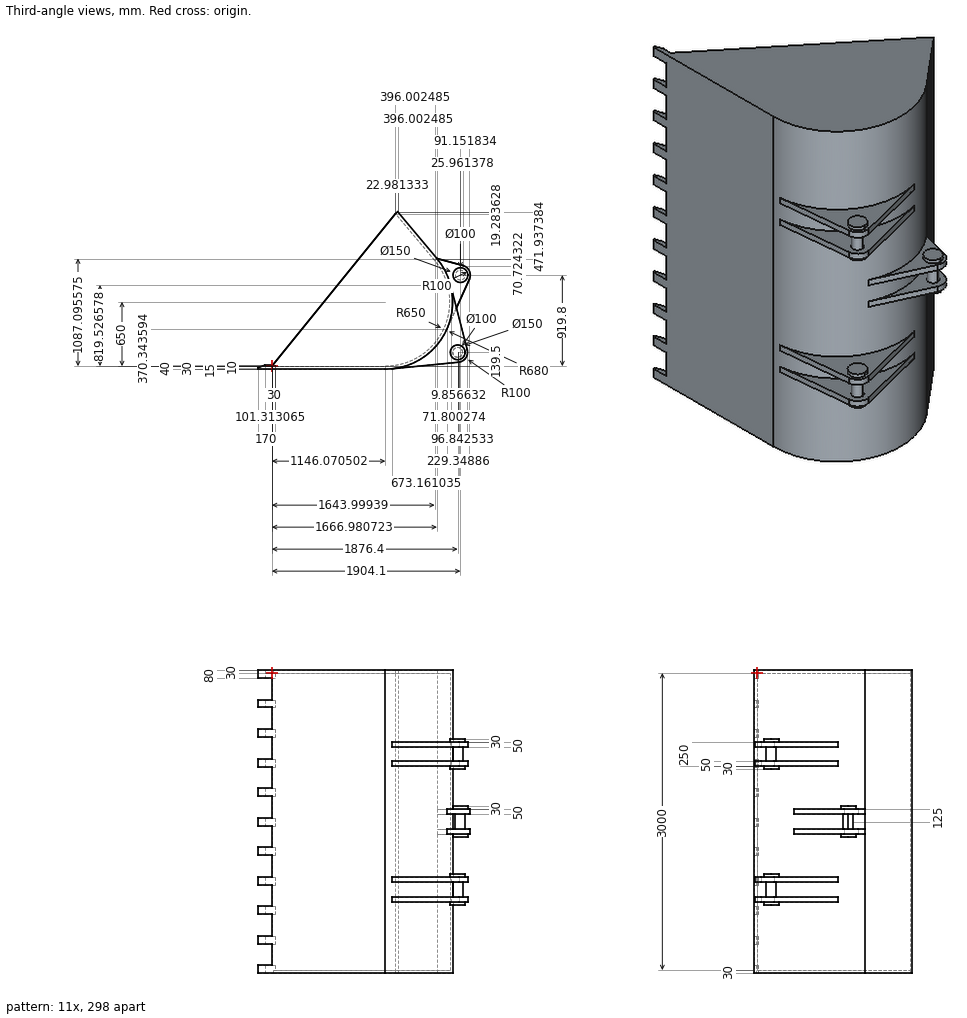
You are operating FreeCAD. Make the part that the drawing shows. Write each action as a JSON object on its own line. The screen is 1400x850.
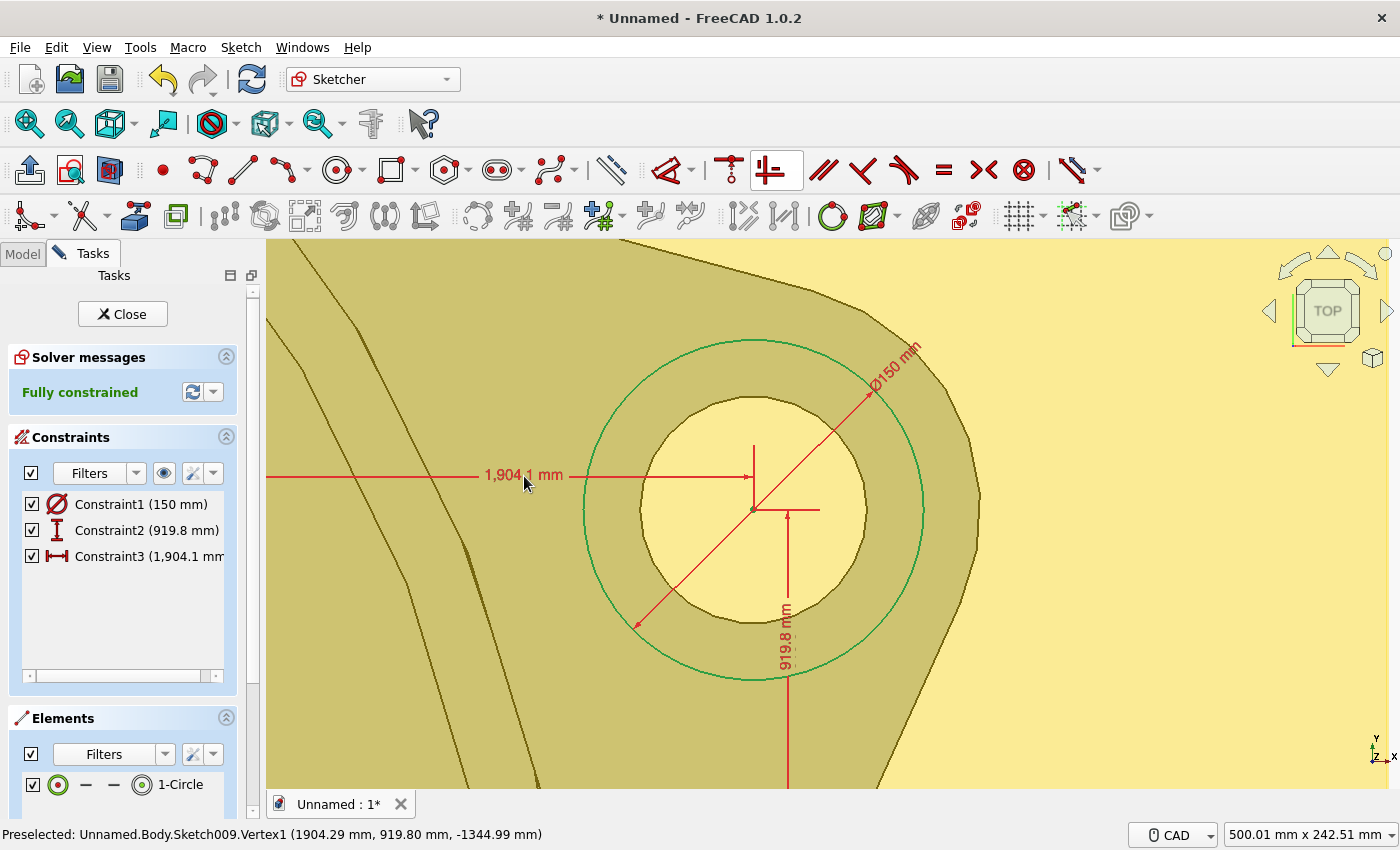
{"action": "left_click", "coordinate": [123, 314]}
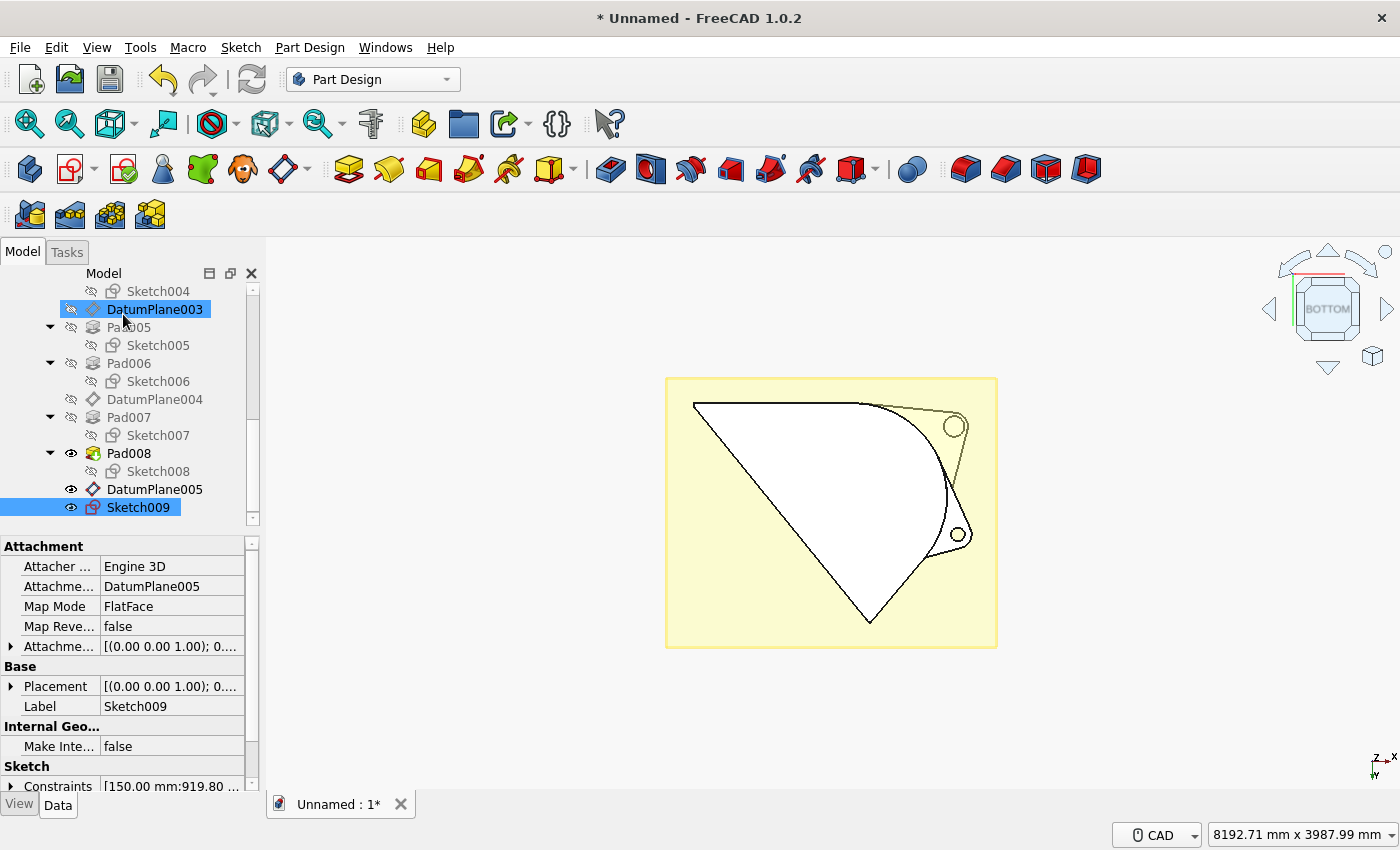
{"action": "left_click", "coordinate": [350, 170]}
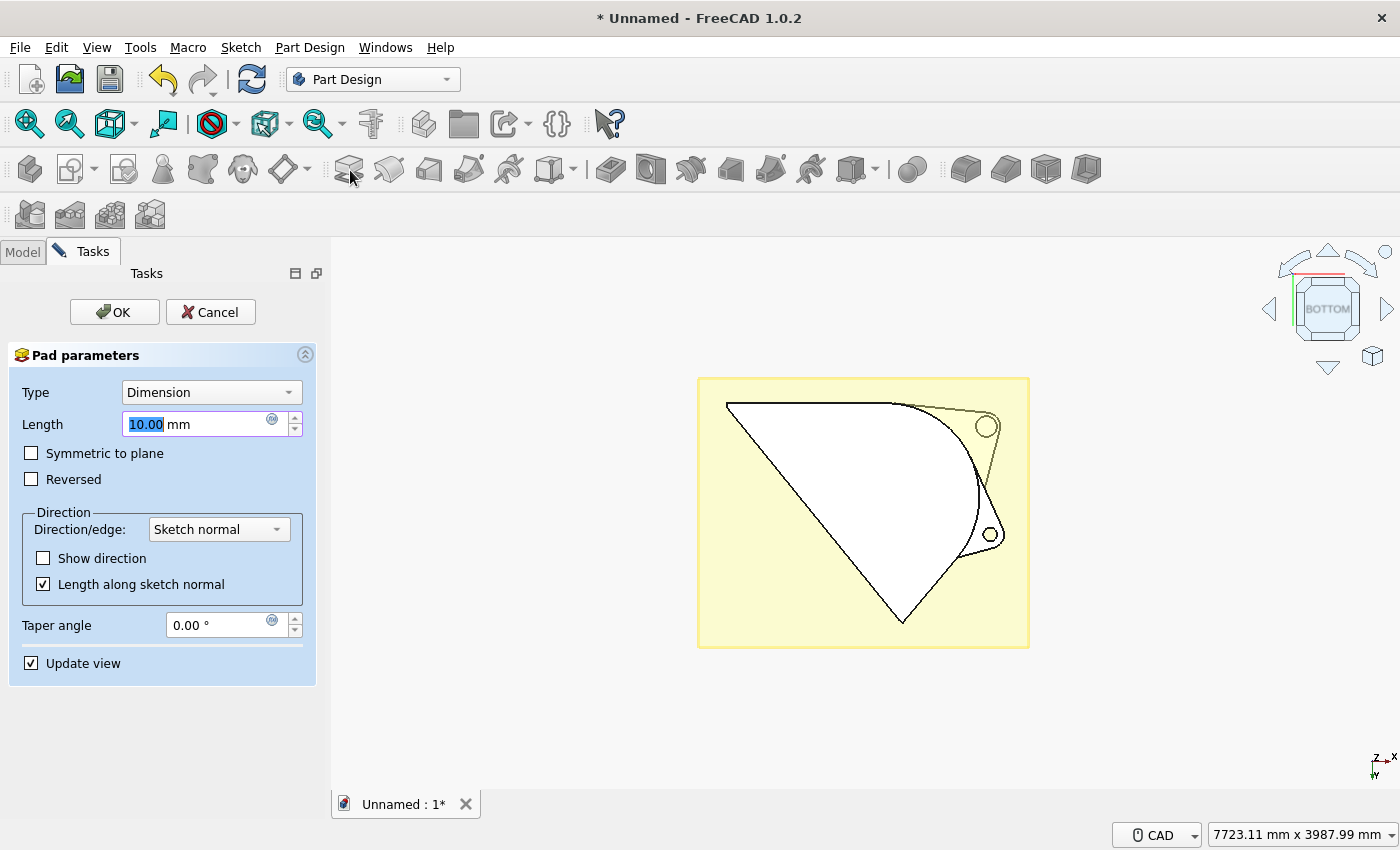
{"action": "type", "text": "30"}
{"action": "key", "text": "Tab"}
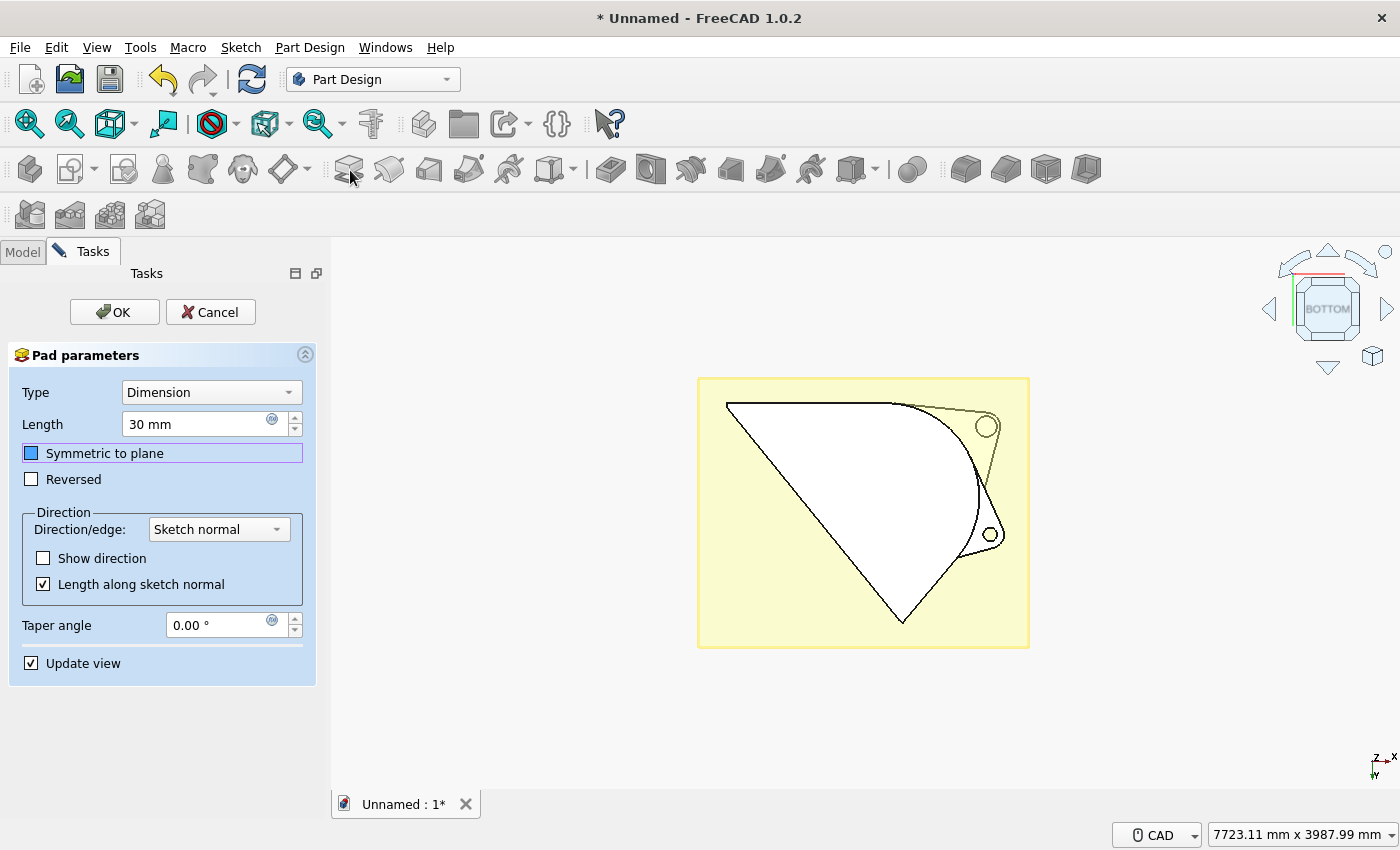
{"action": "left_click", "coordinate": [30, 479]}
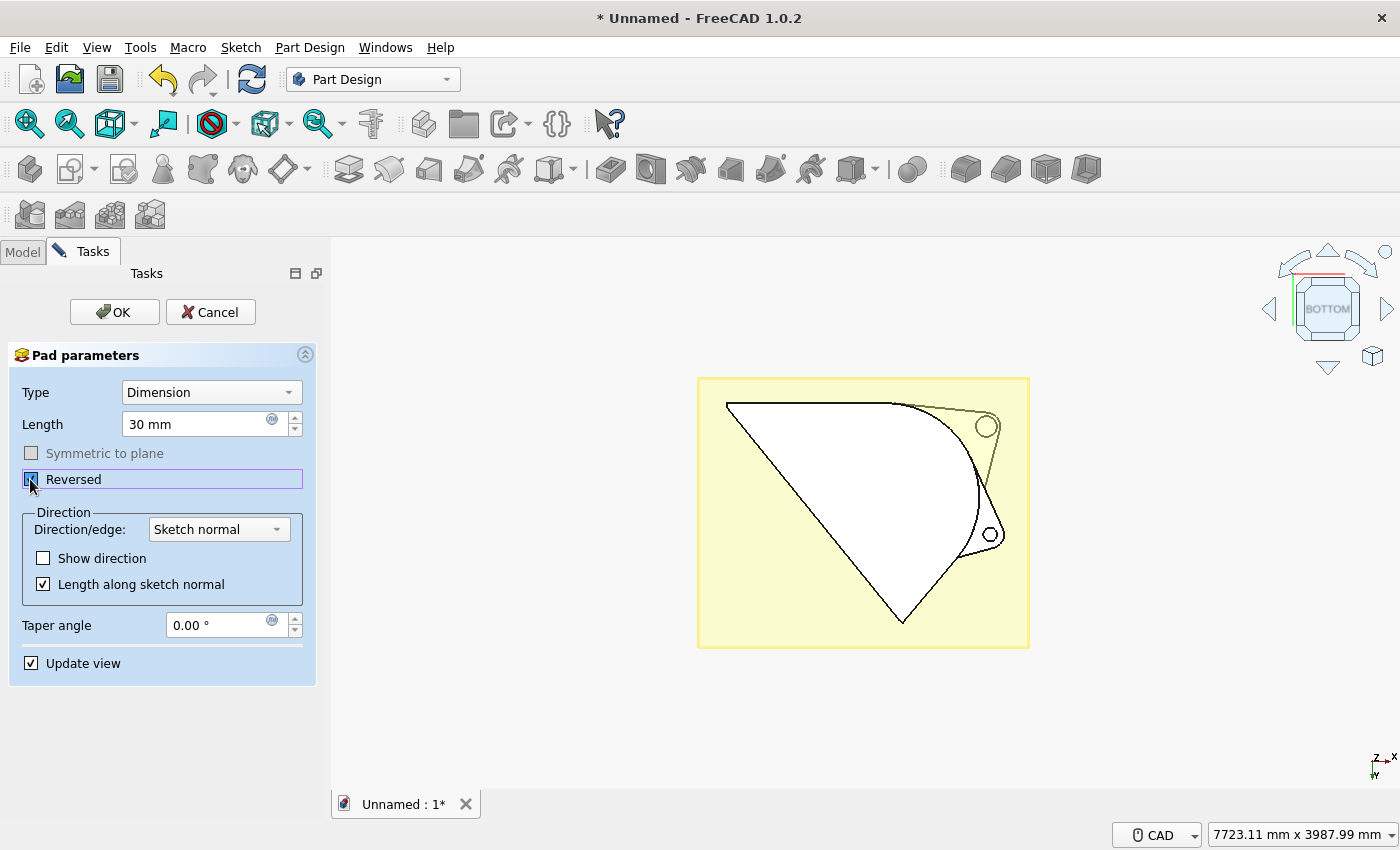
{"action": "left_click", "coordinate": [115, 312]}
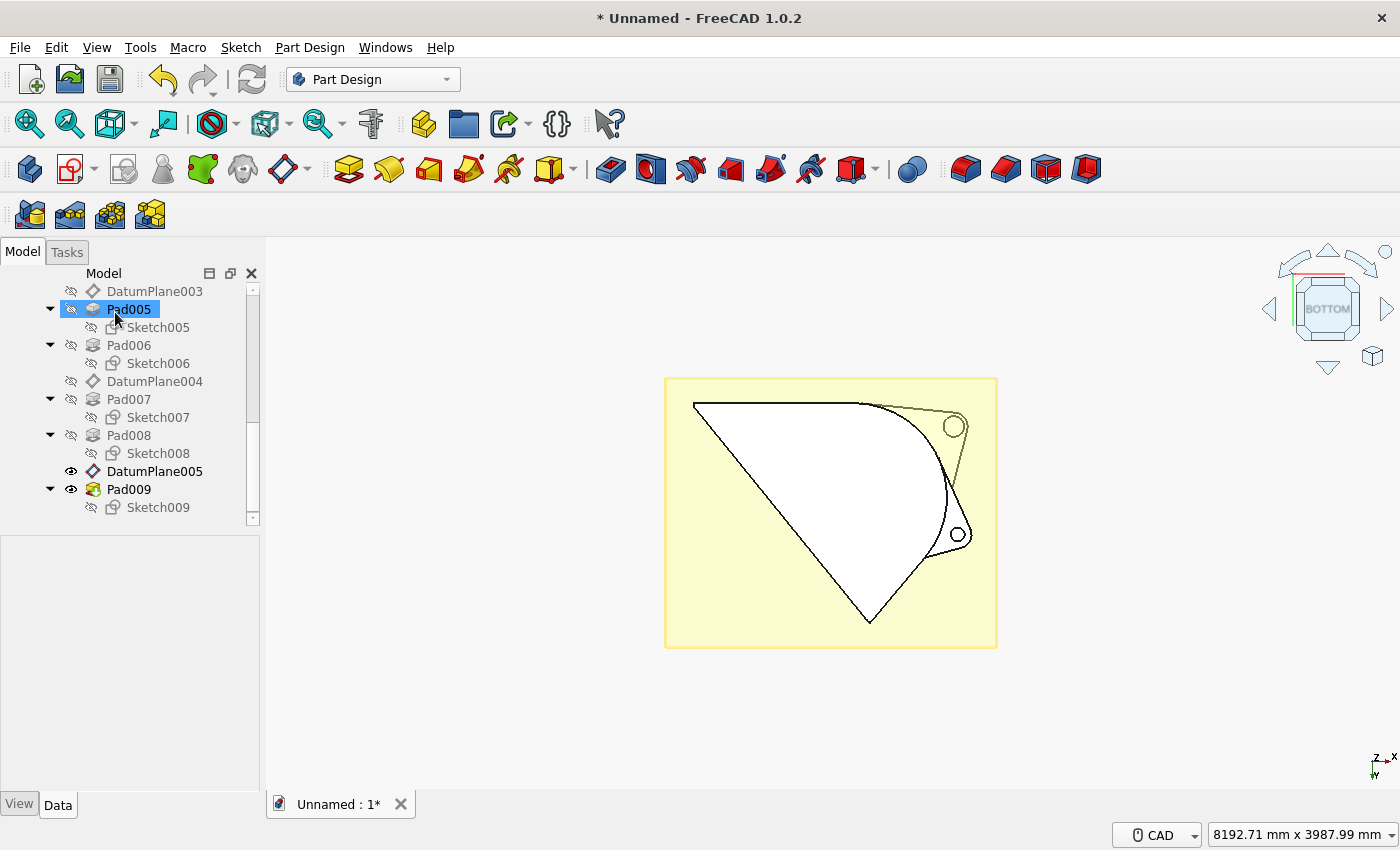
{"action": "left_click", "coordinate": [116, 471]}
{"action": "key", "text": "space"}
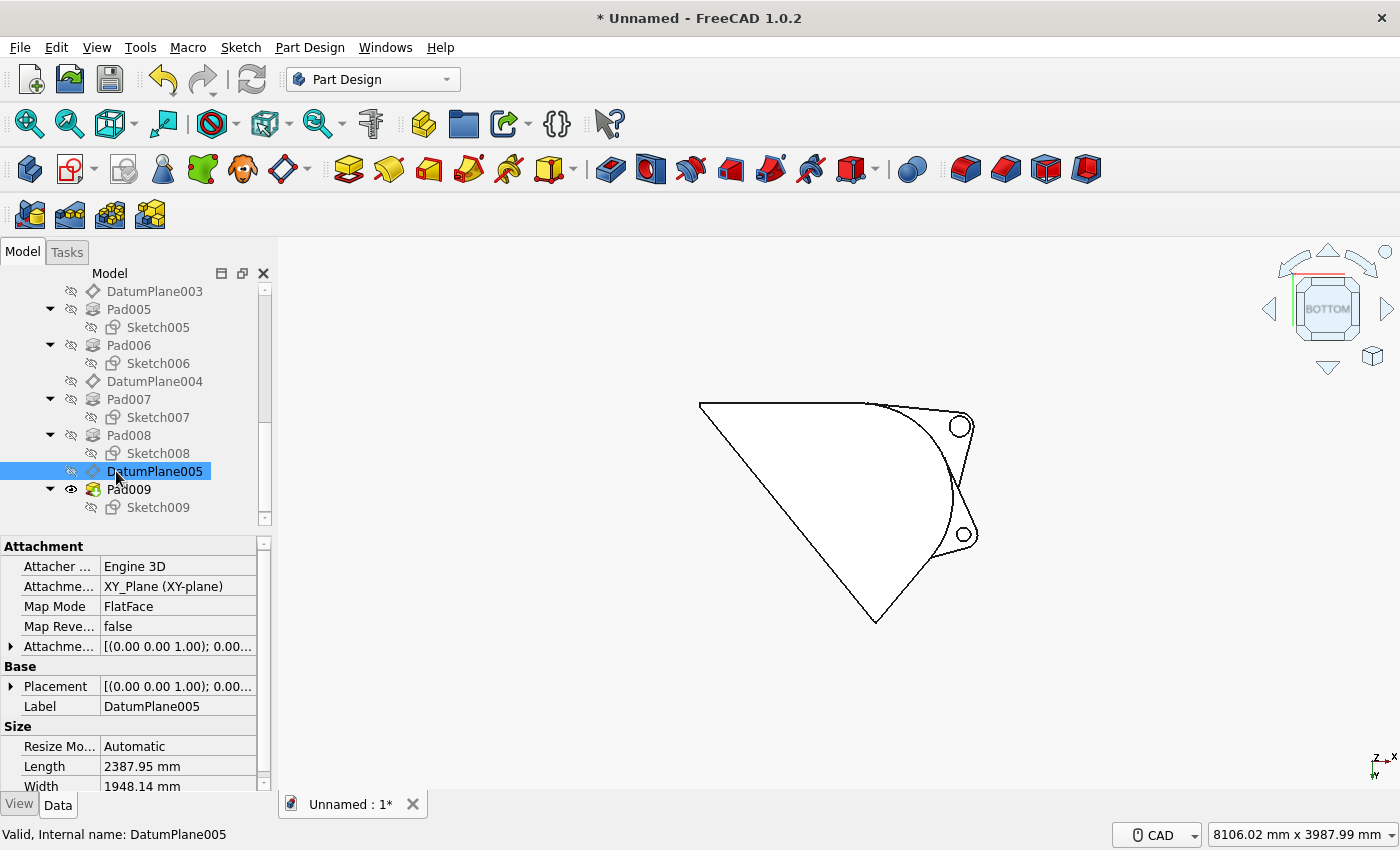
{"action": "left_click", "coordinate": [30, 124]}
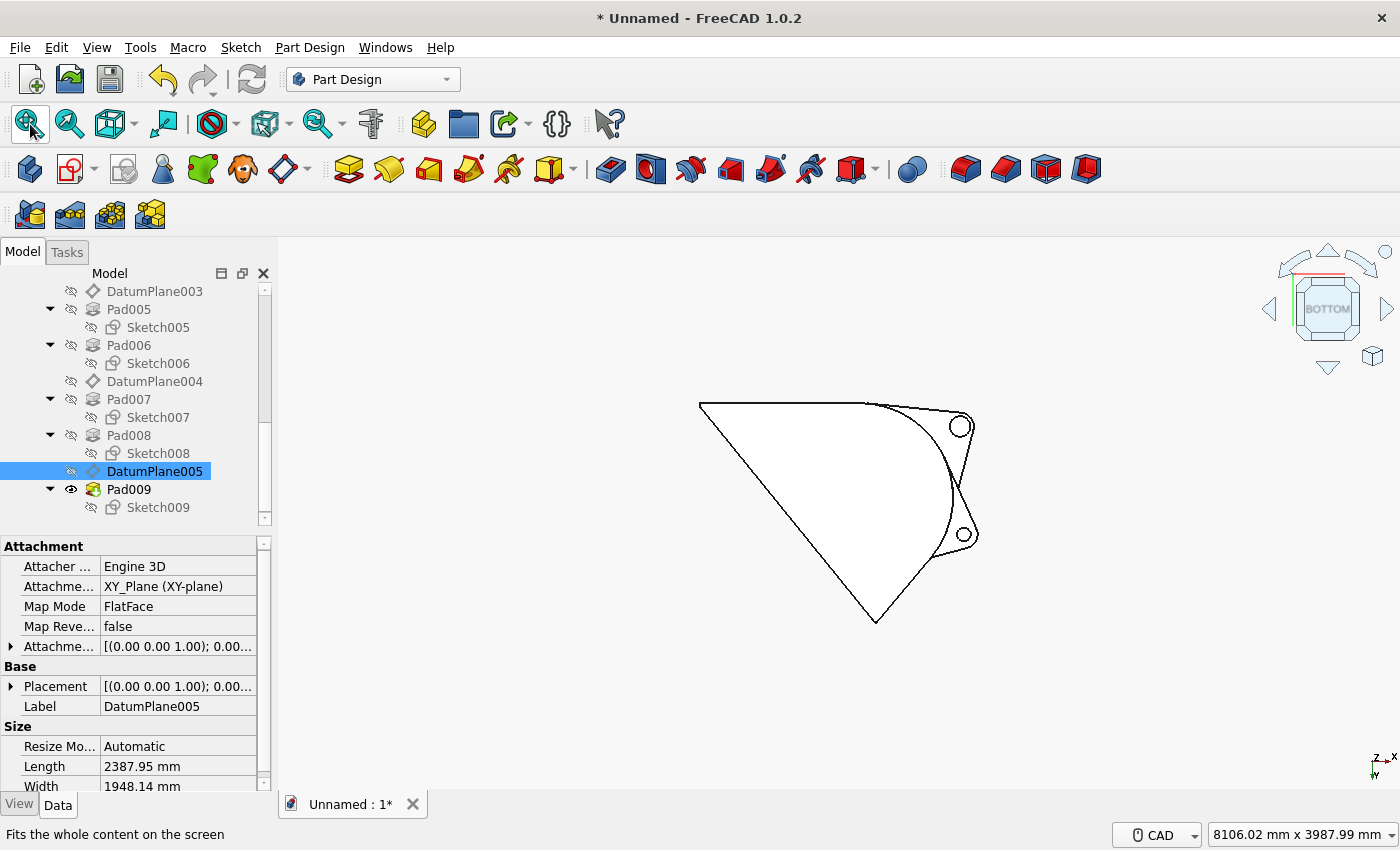
{"action": "key", "text": "0"}